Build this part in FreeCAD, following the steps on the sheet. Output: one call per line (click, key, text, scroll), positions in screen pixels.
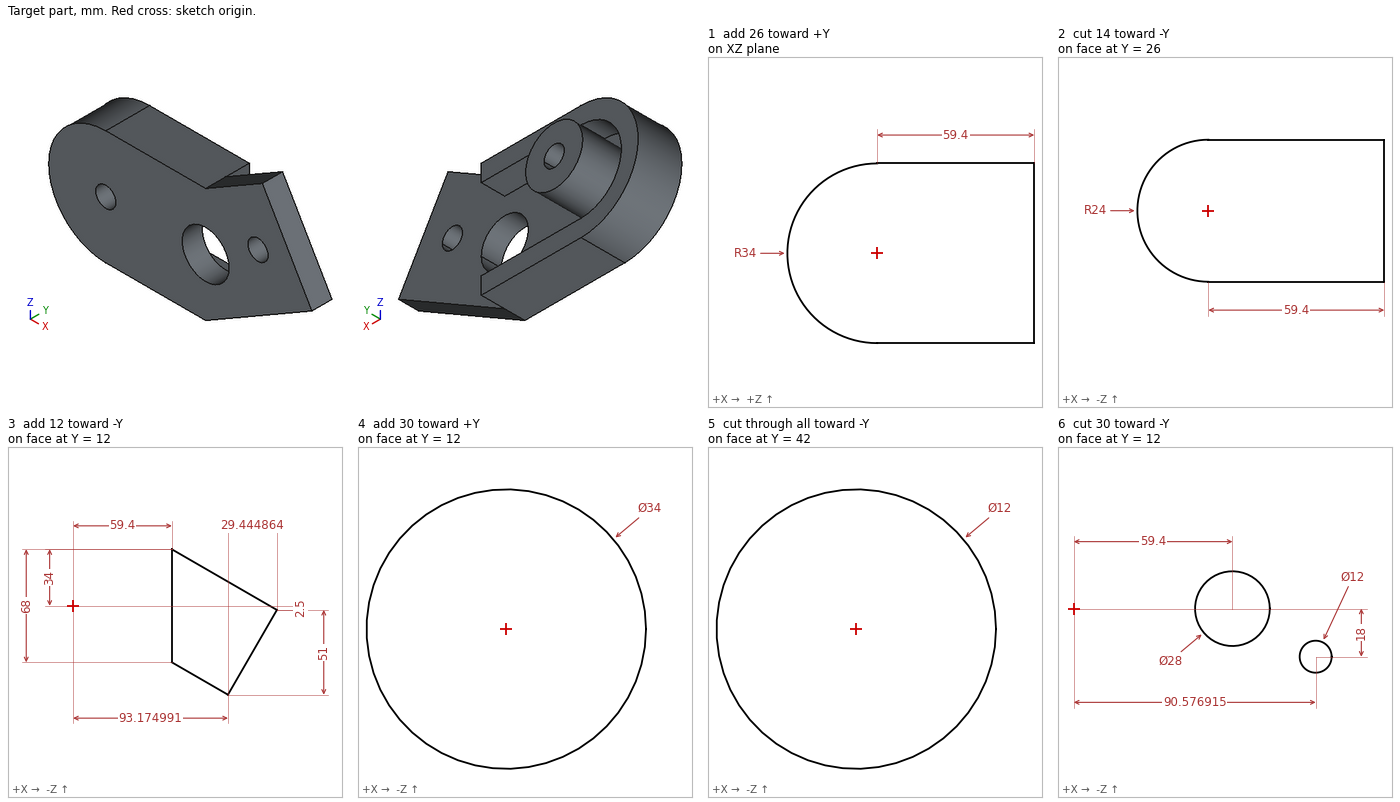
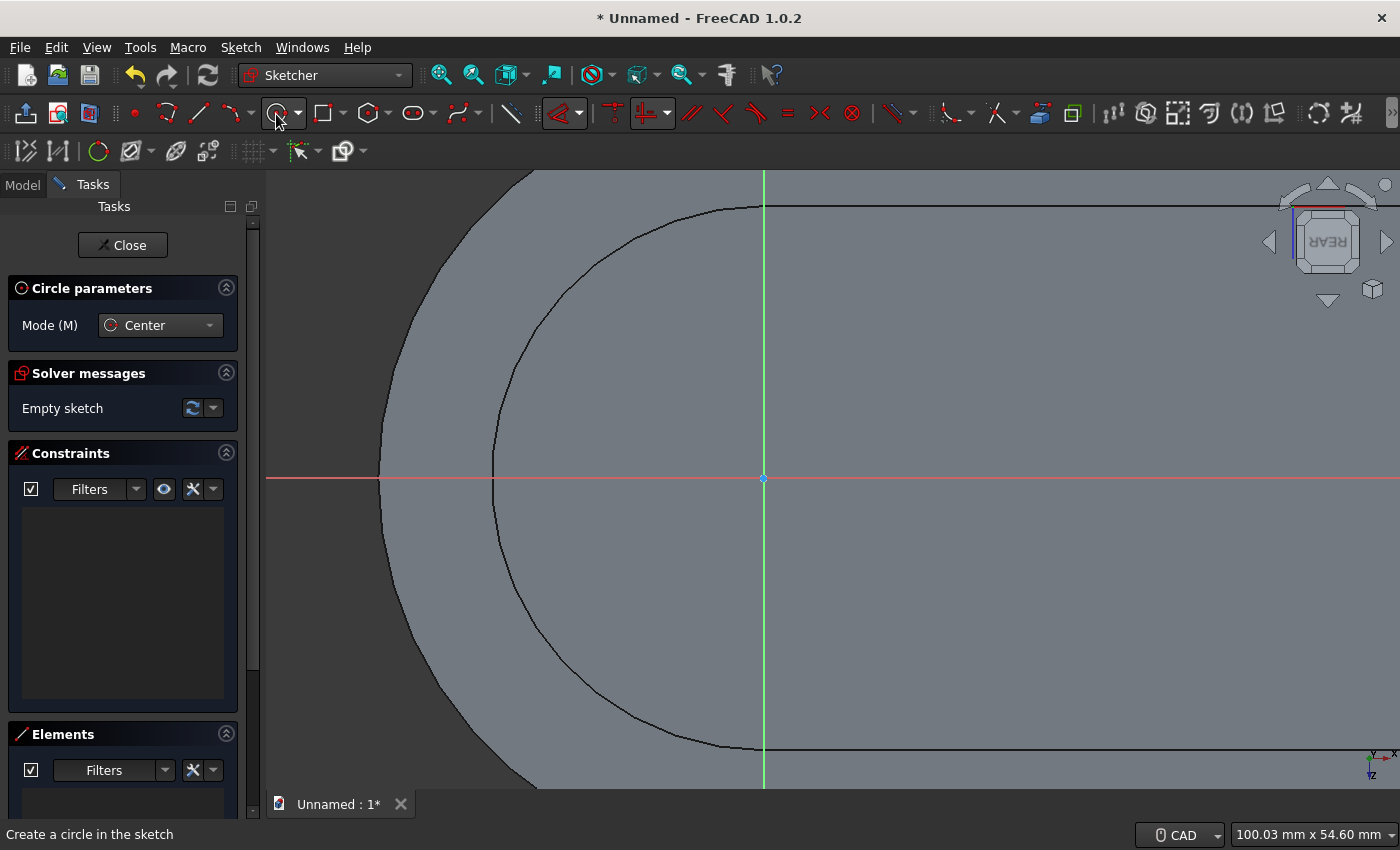
click(764, 478)
move(900, 342)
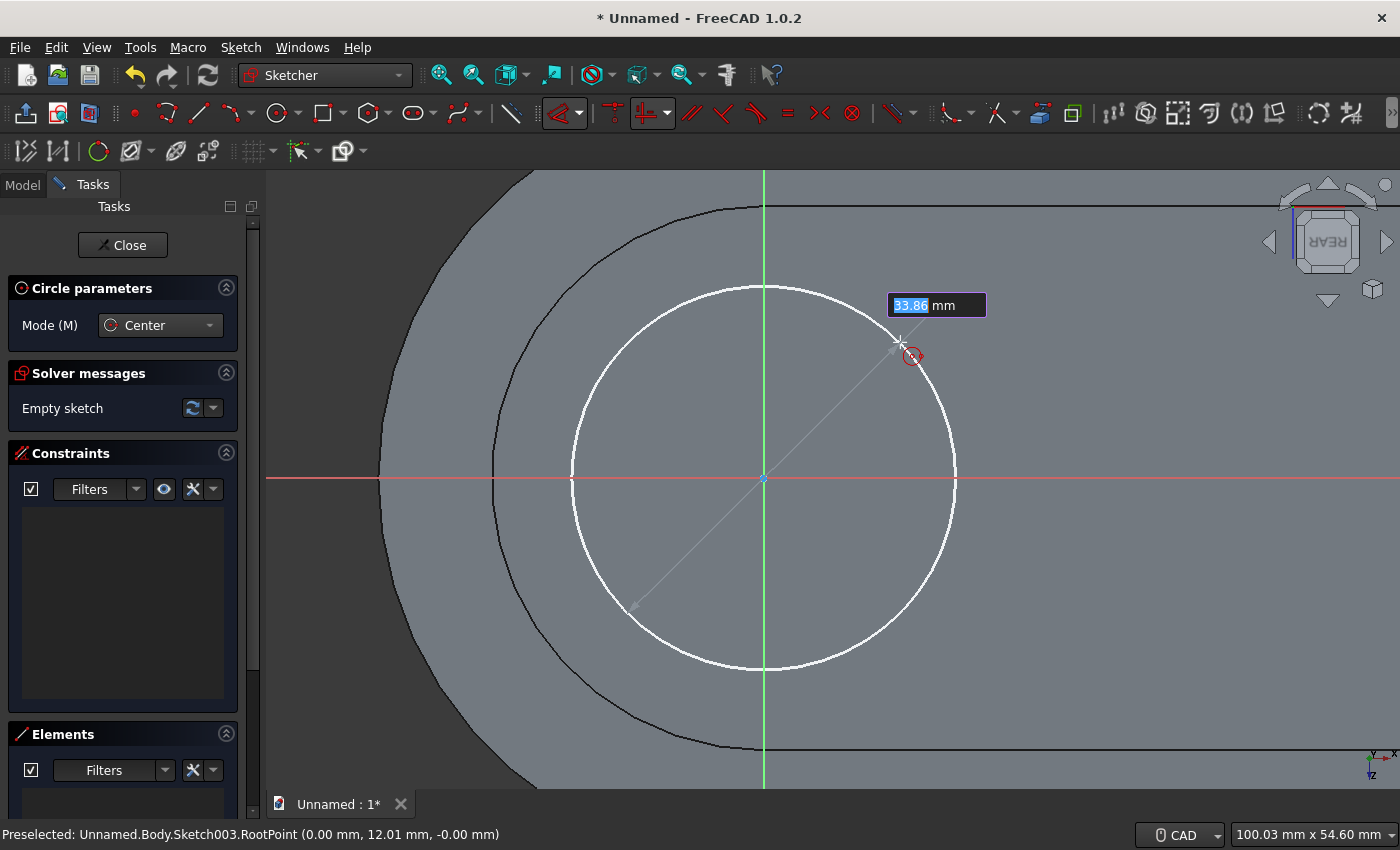
text(34)
key(Return)
key(Escape)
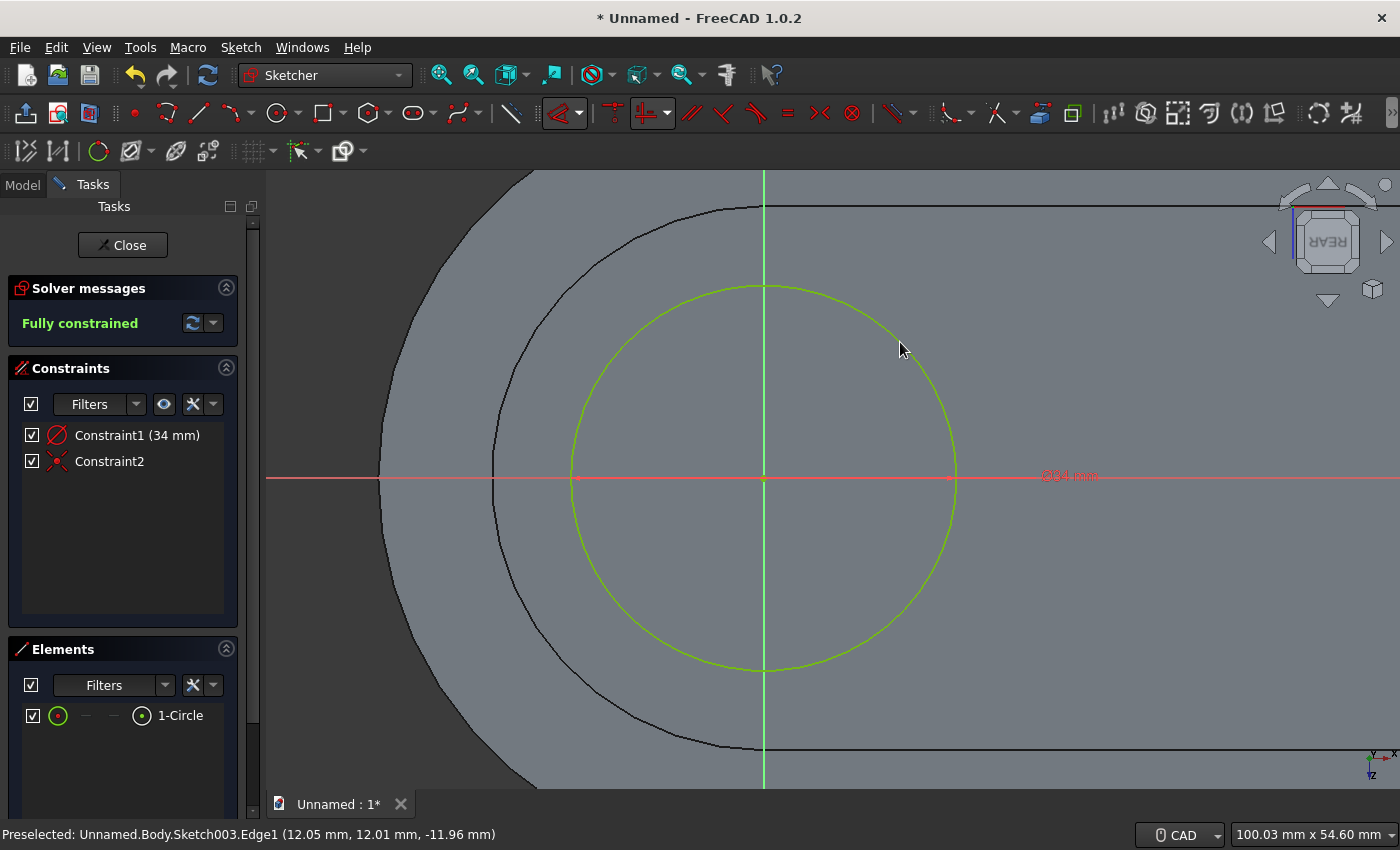
click(123, 245)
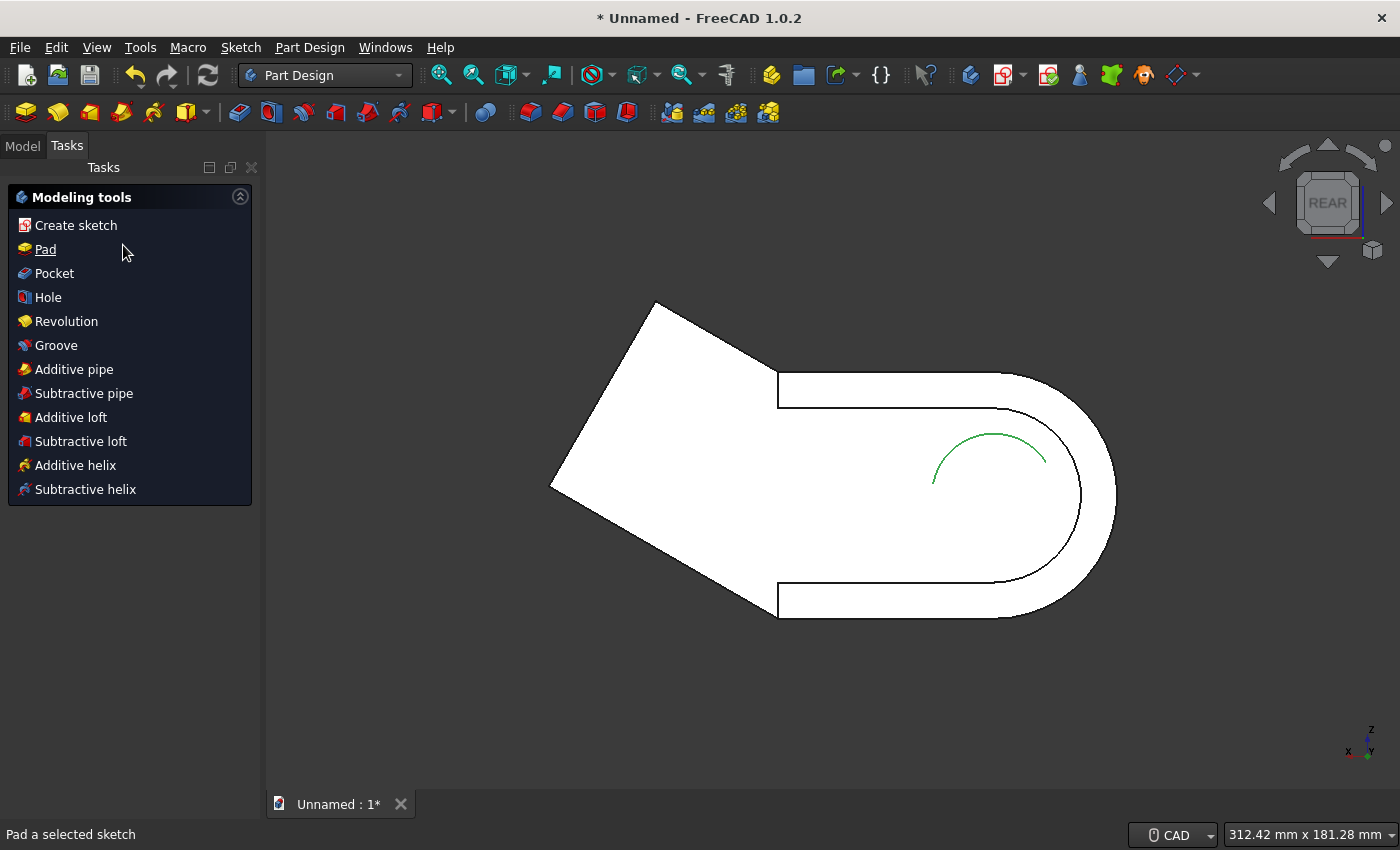
click(26, 112)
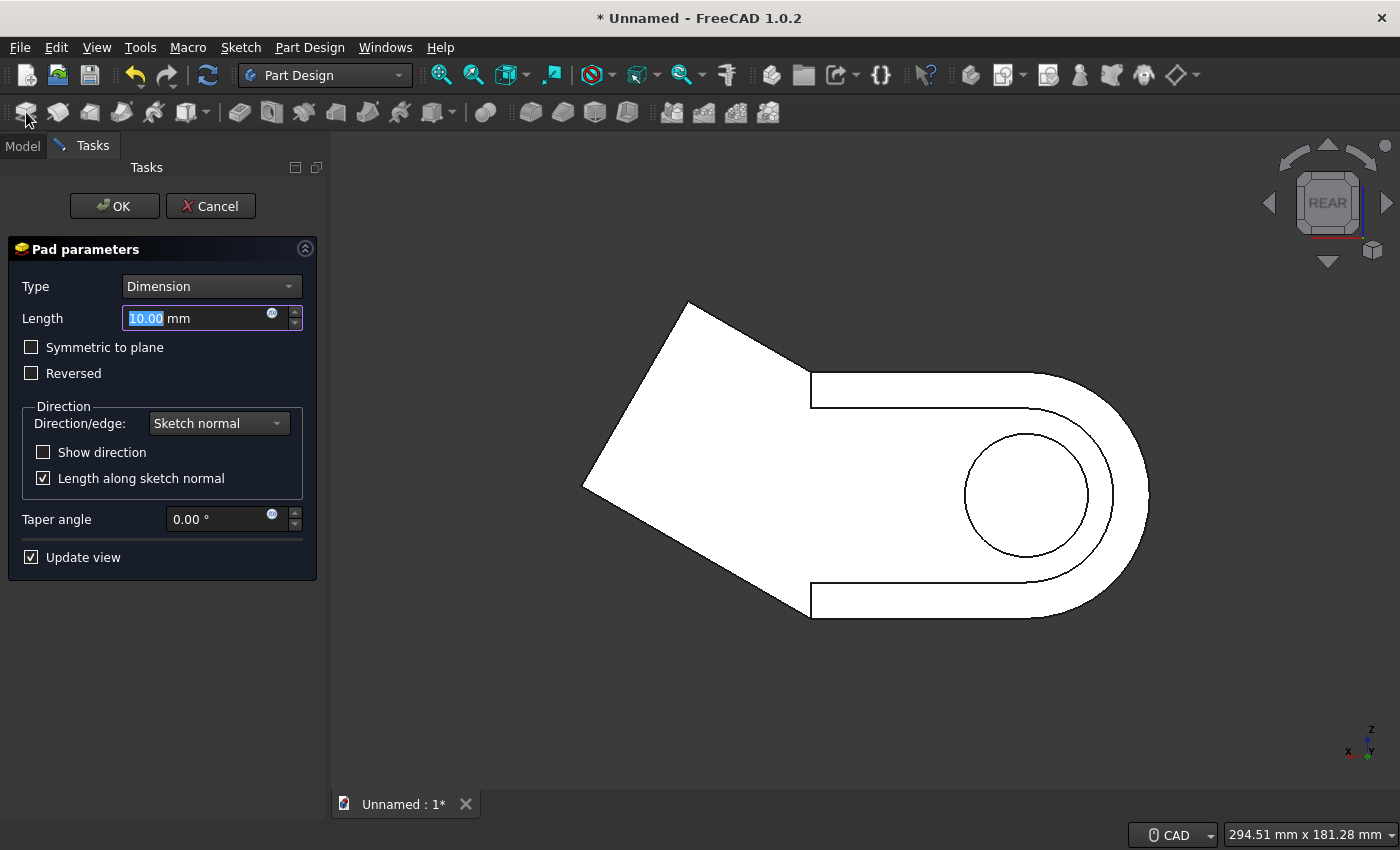
text(30)
key(Tab)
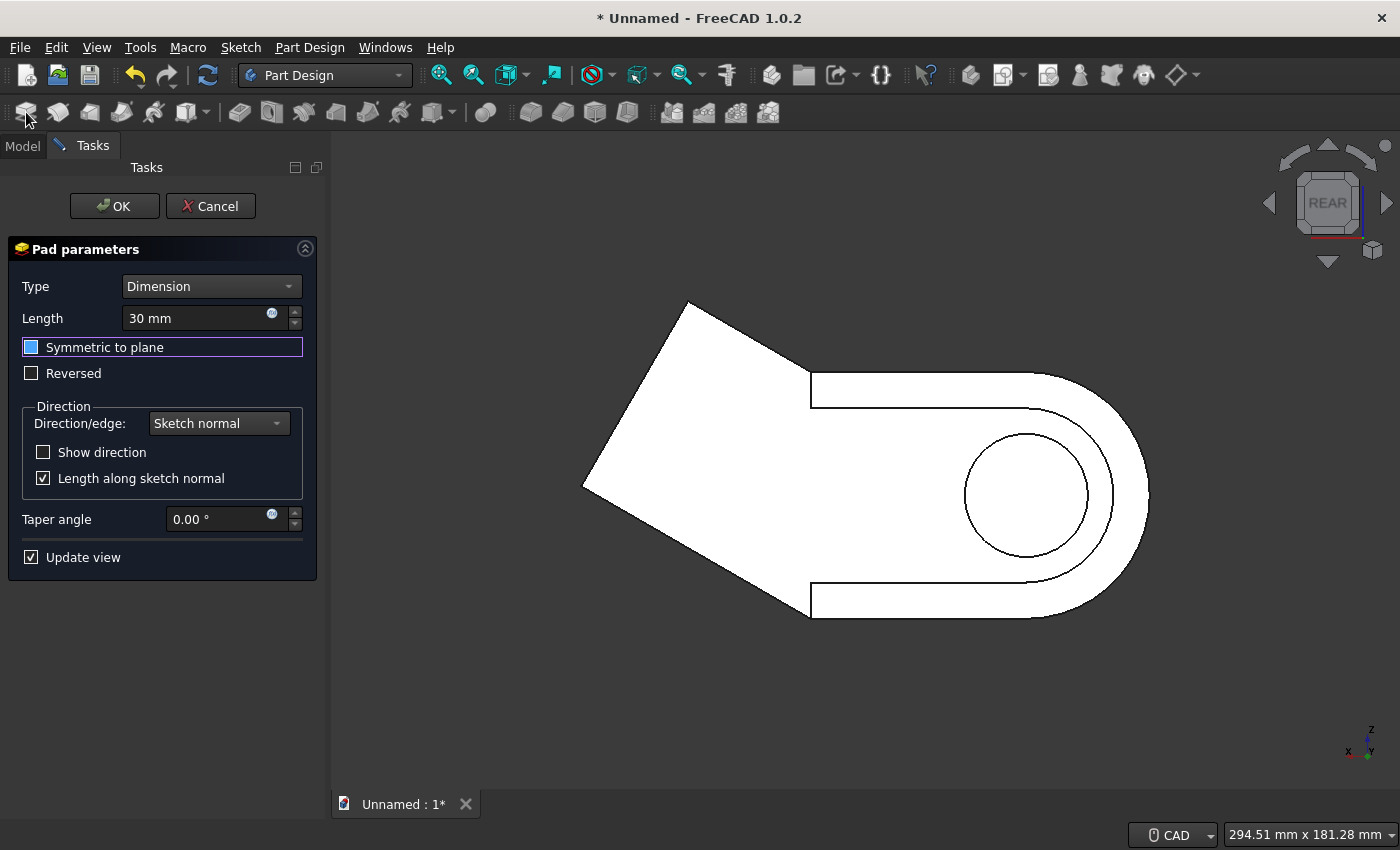
click(115, 206)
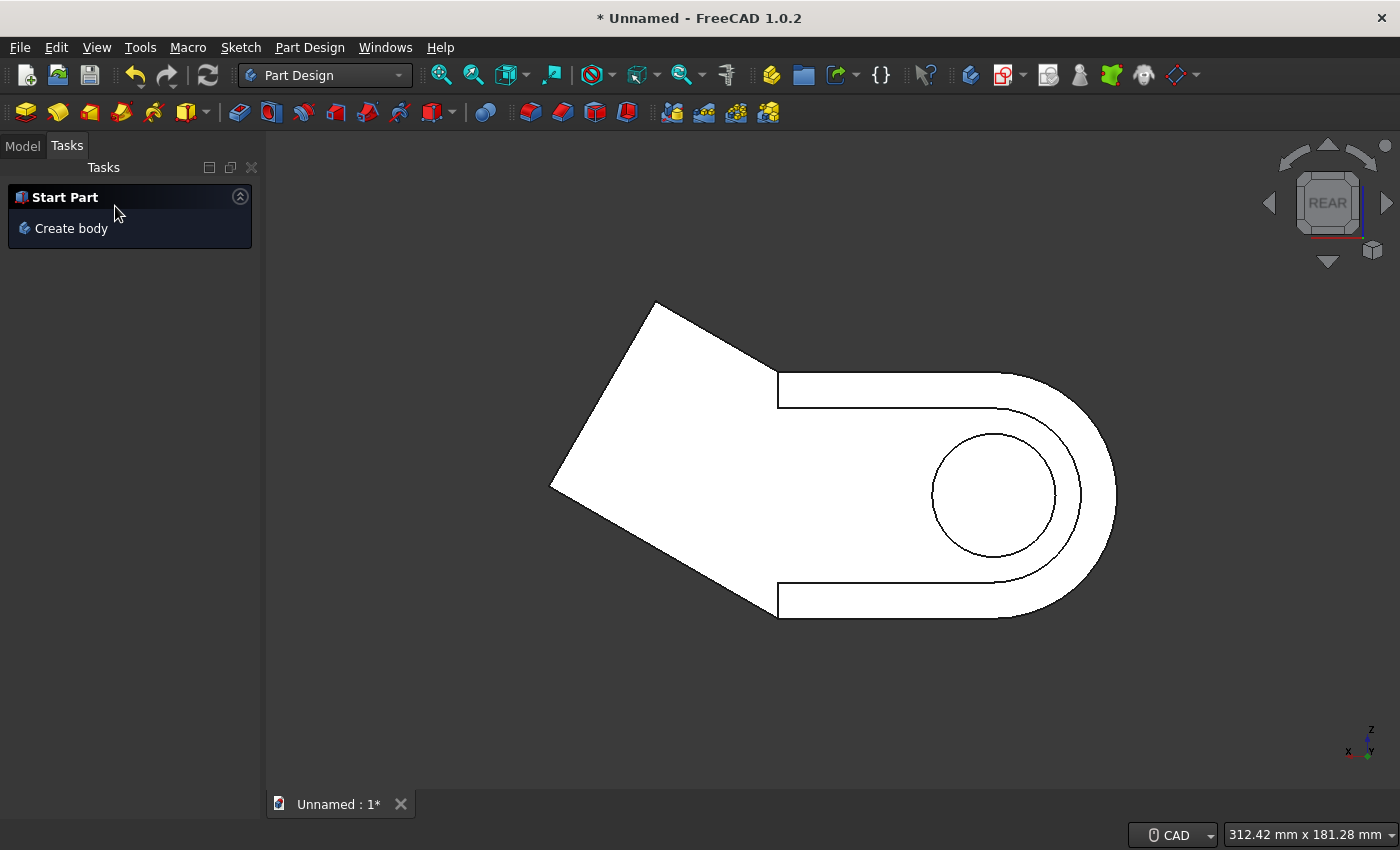
click(994, 494)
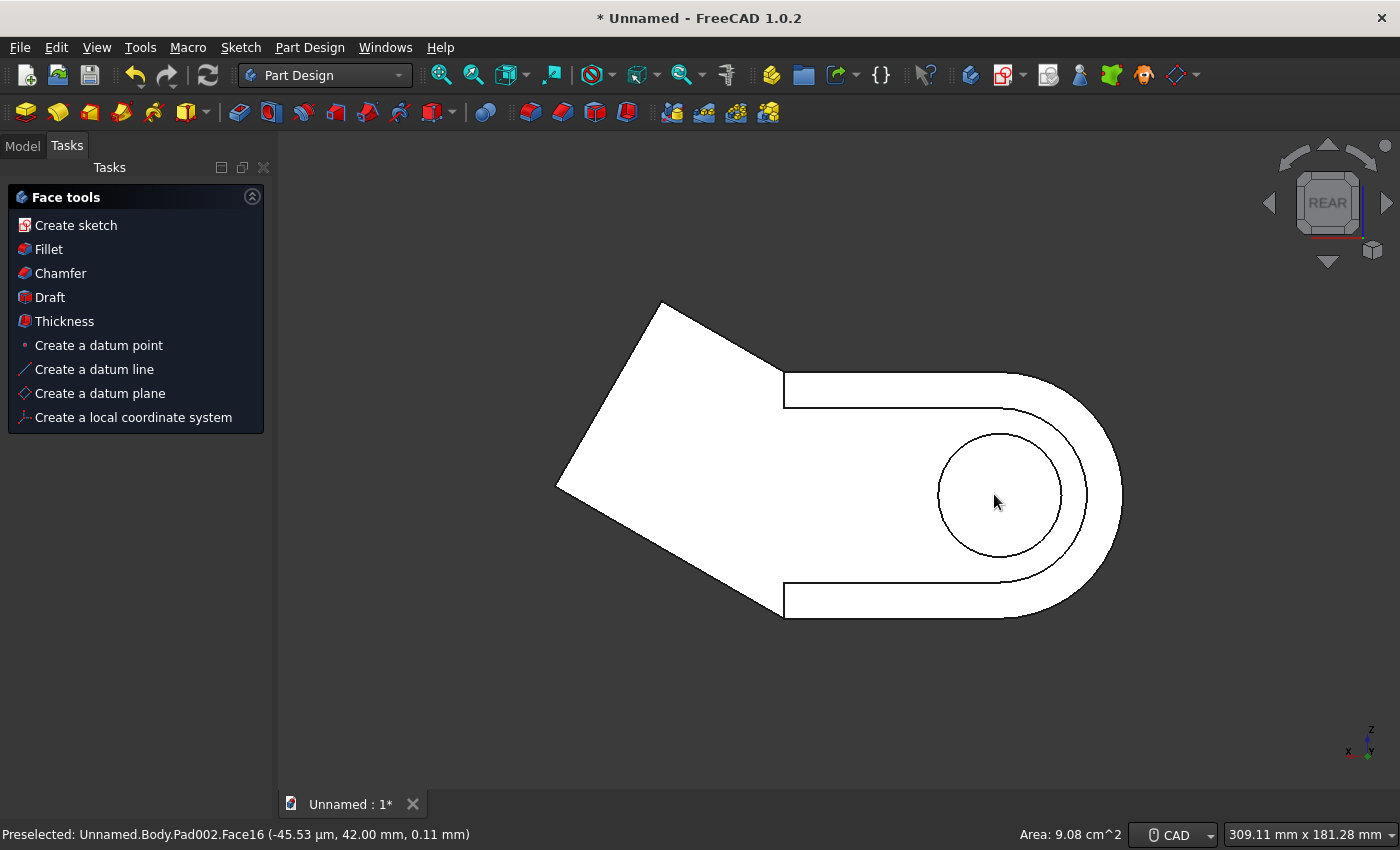
click(1004, 76)